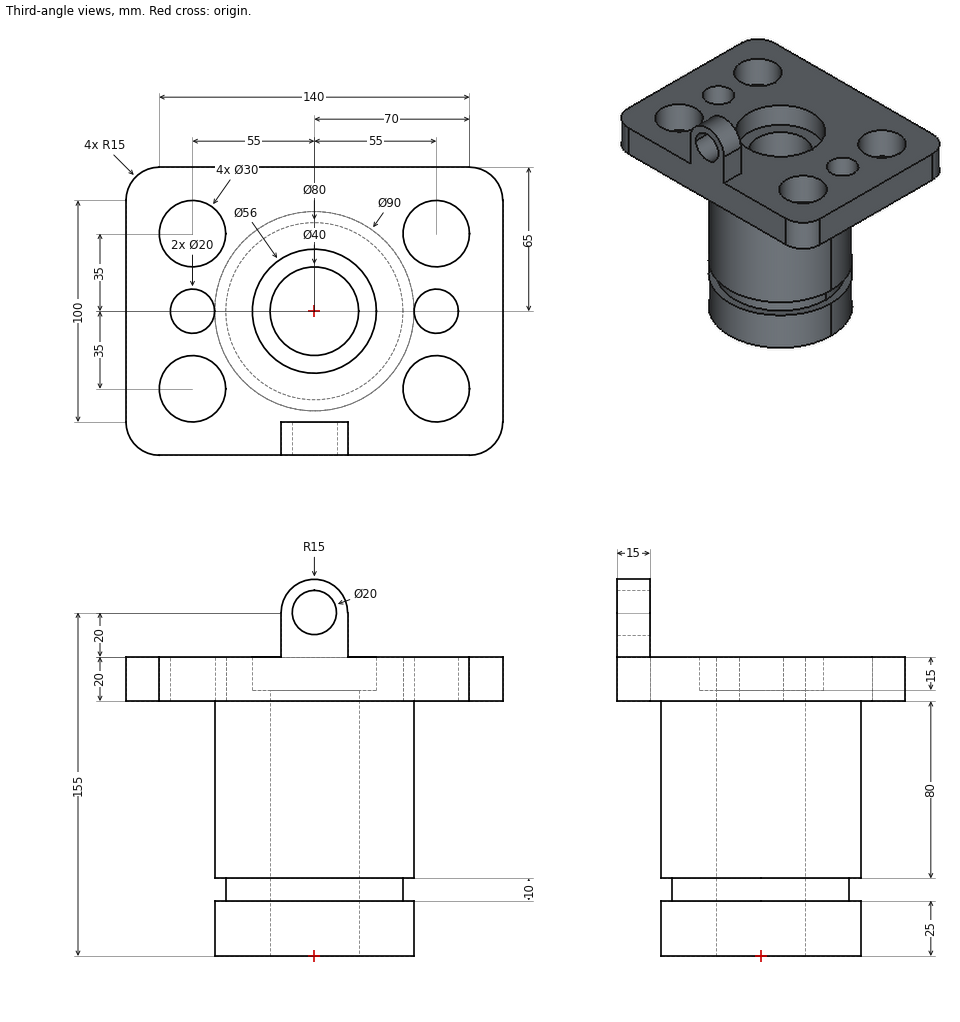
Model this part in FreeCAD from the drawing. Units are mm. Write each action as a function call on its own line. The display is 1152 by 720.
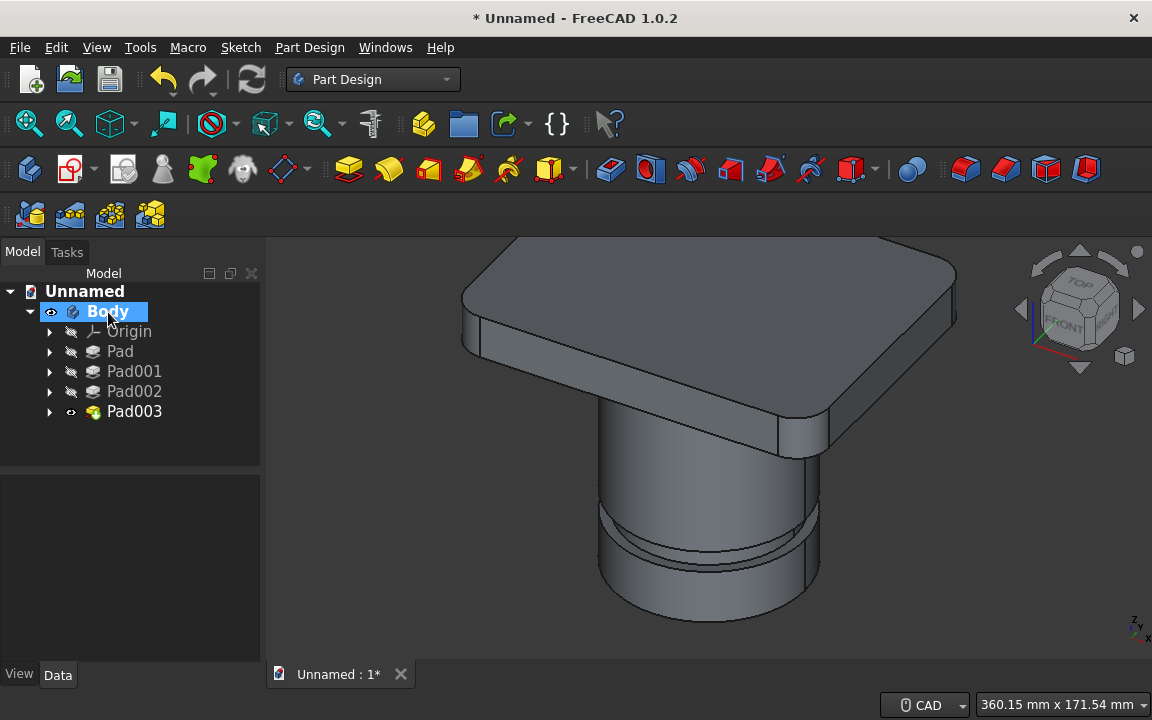
click(30, 124)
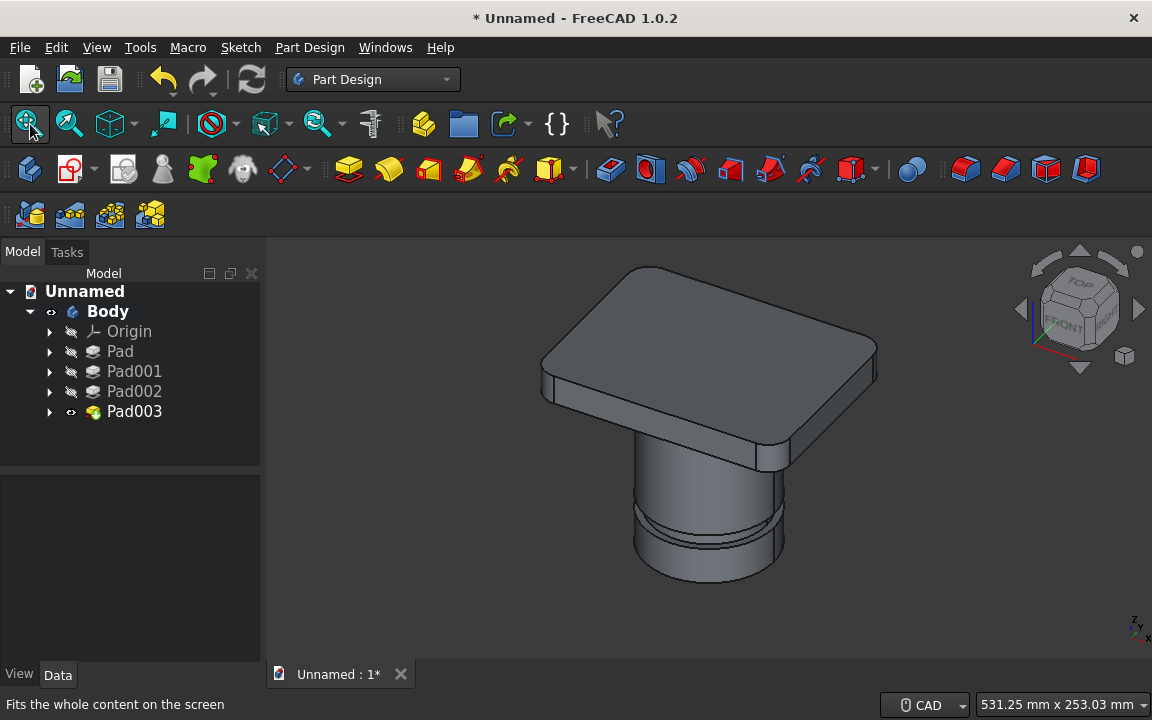
click(709, 355)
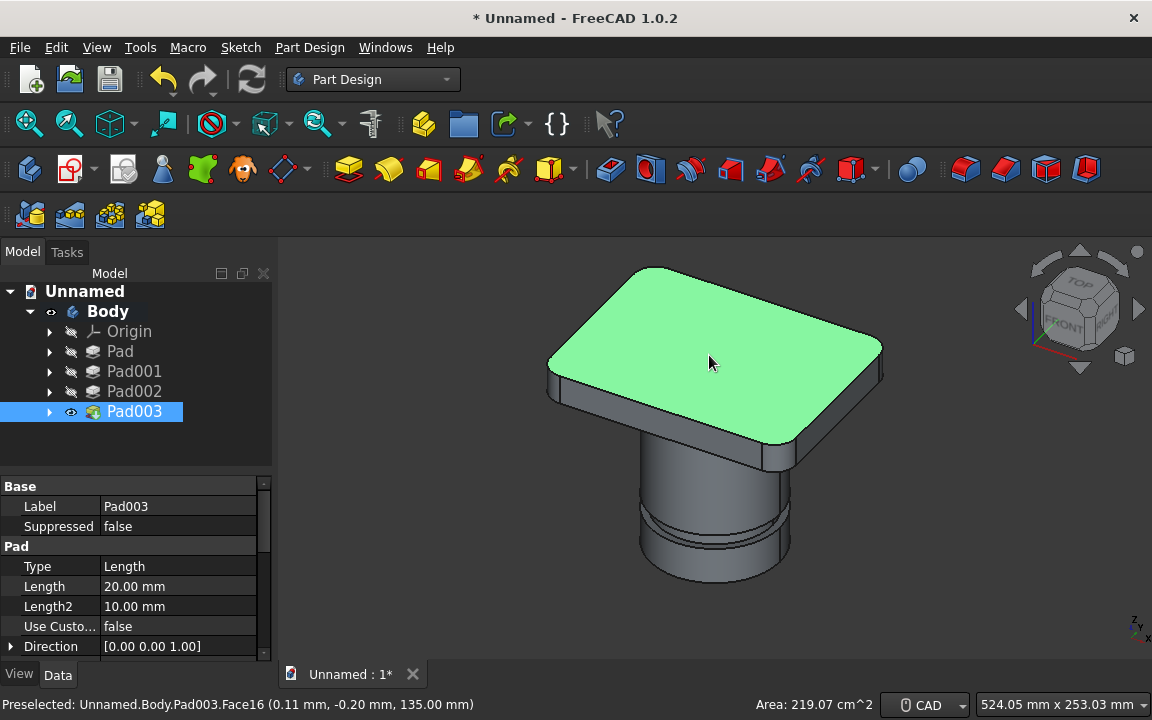
click(70, 170)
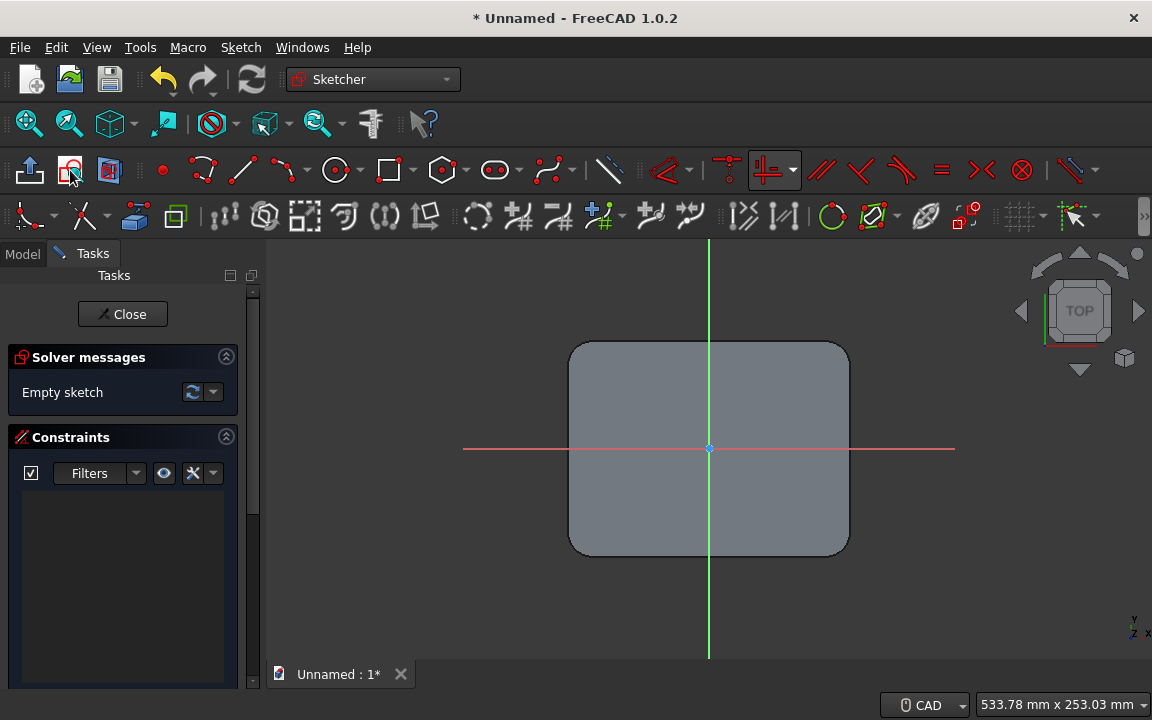
scroll(749, 449, up, 5)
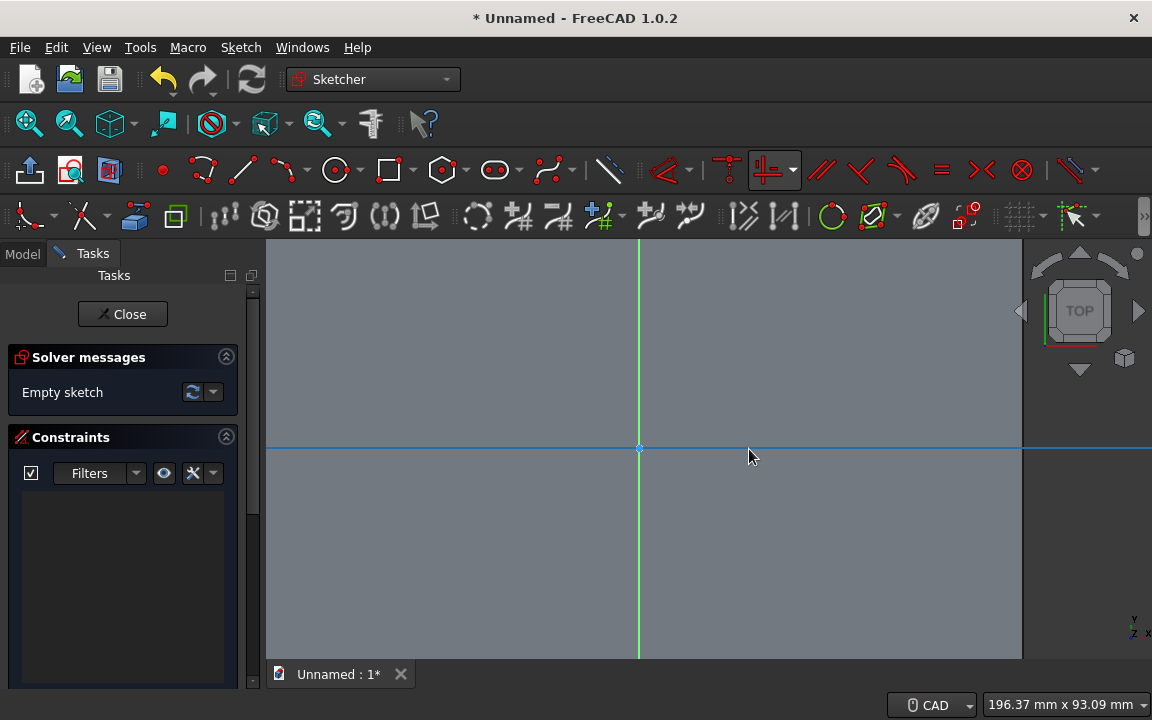
click(336, 170)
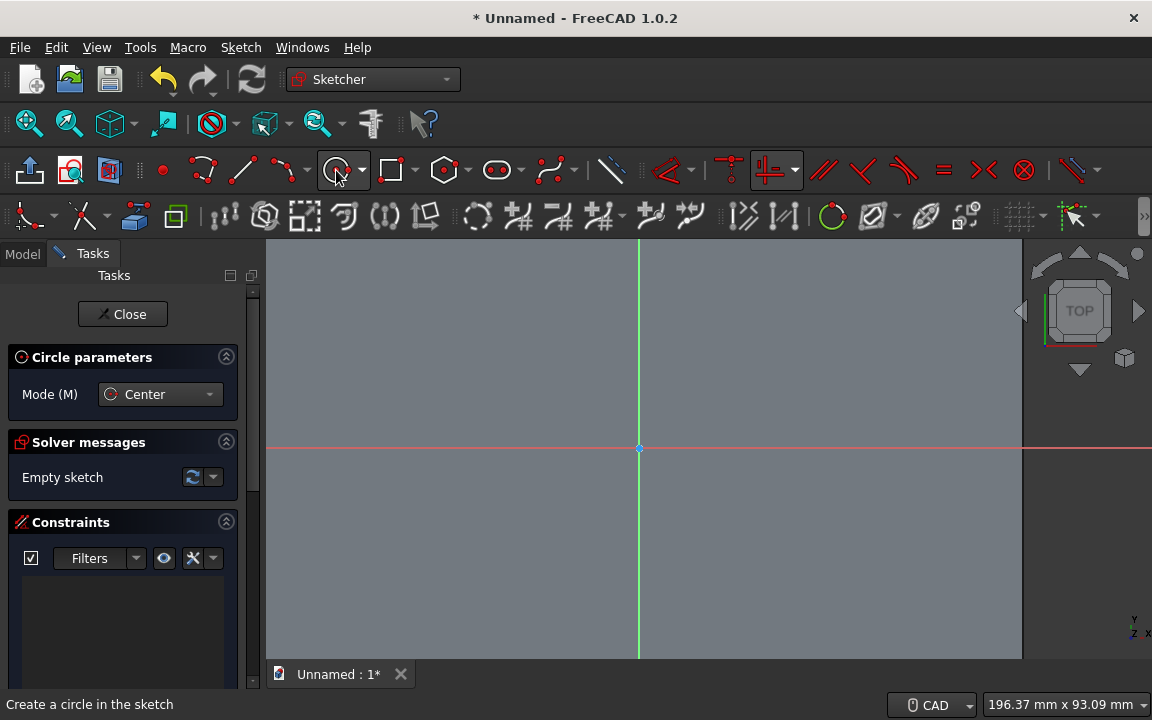
click(639, 448)
click(729, 359)
key(Escape)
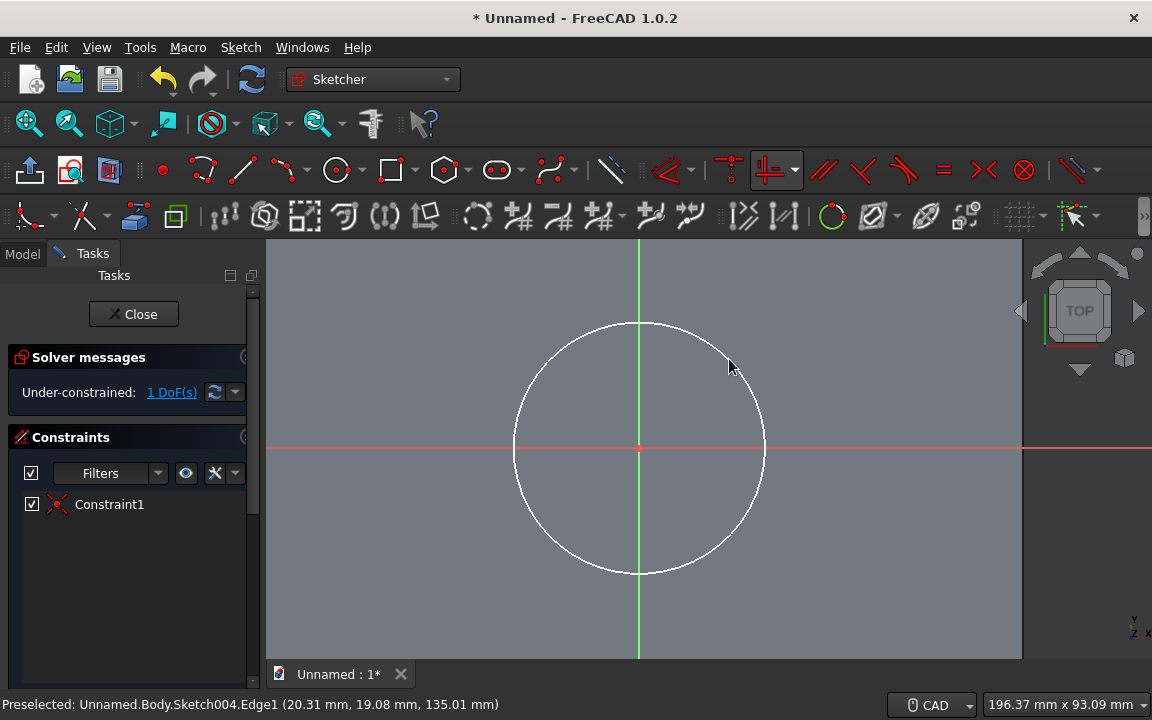
click(666, 170)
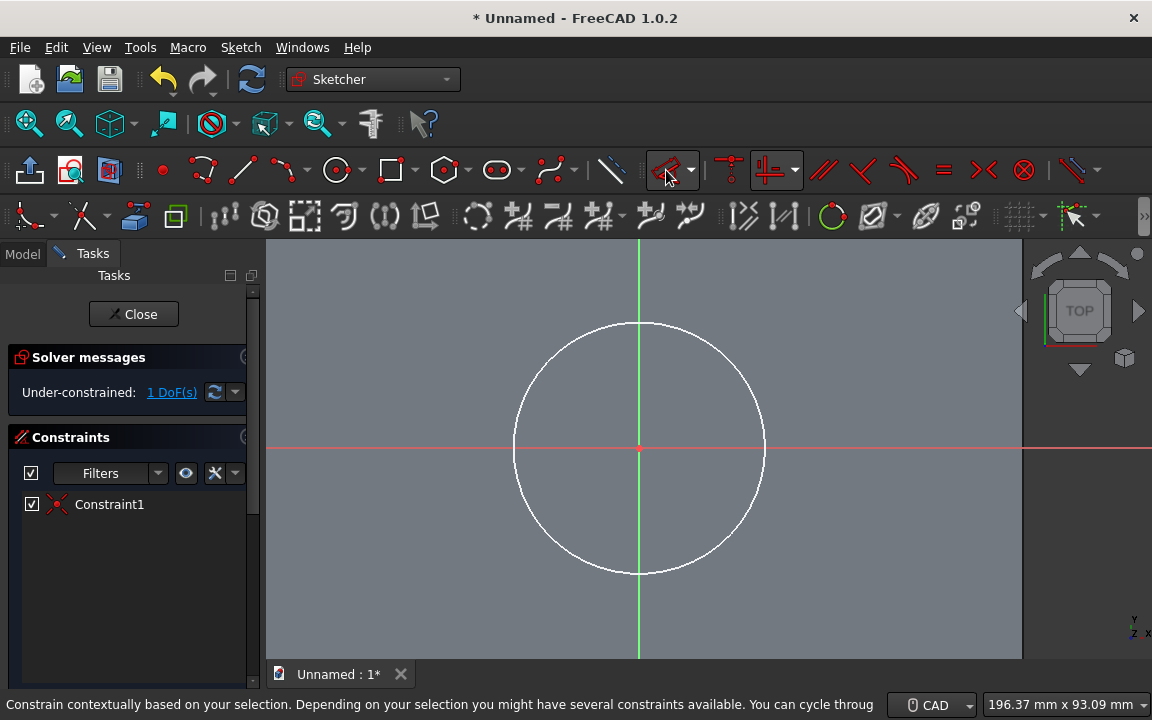
click(728, 359)
click(751, 336)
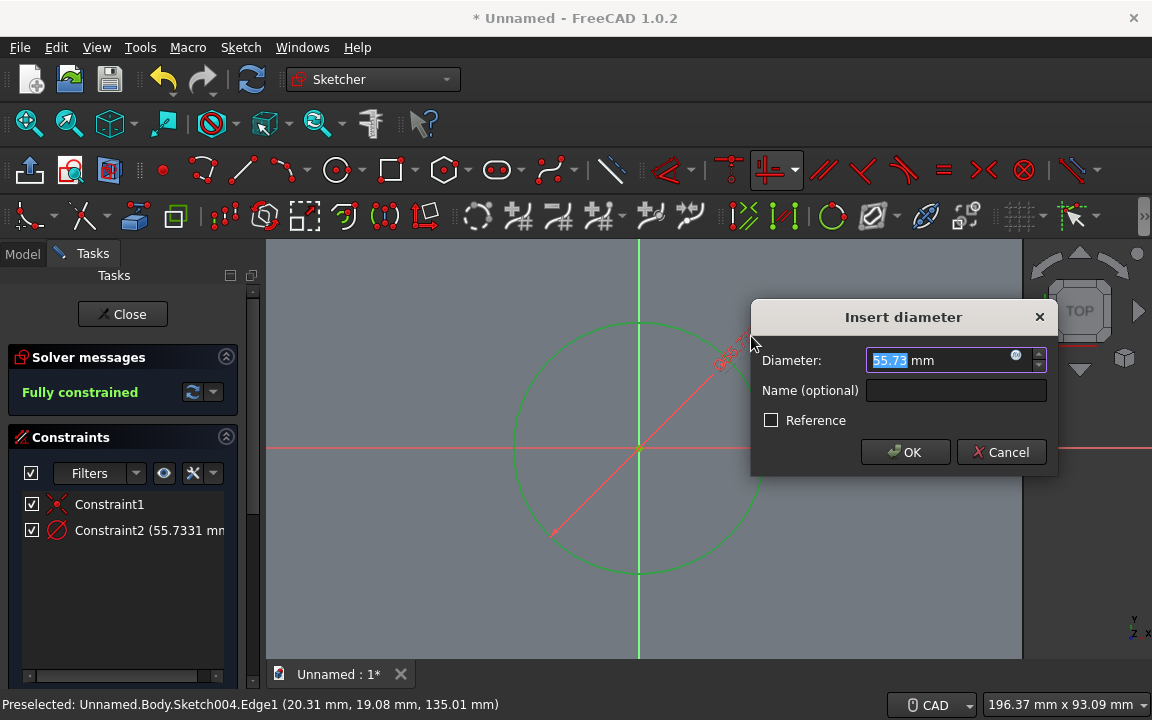
text(56)
key(Return)
key(Escape)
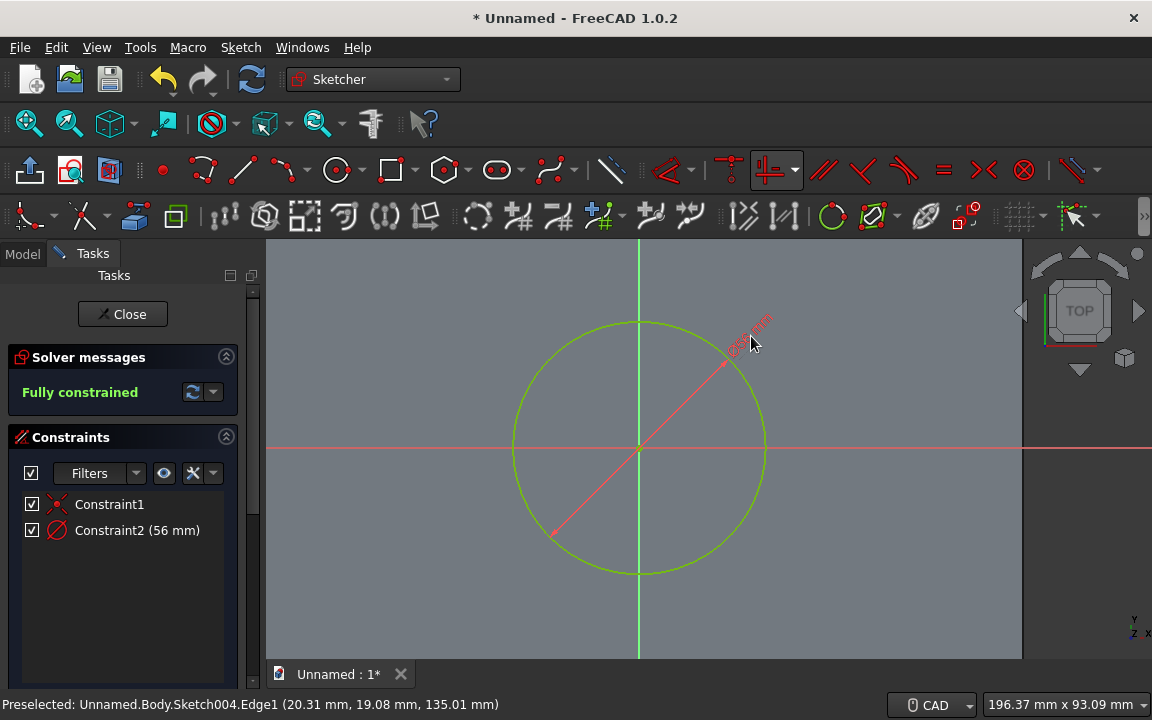
click(123, 314)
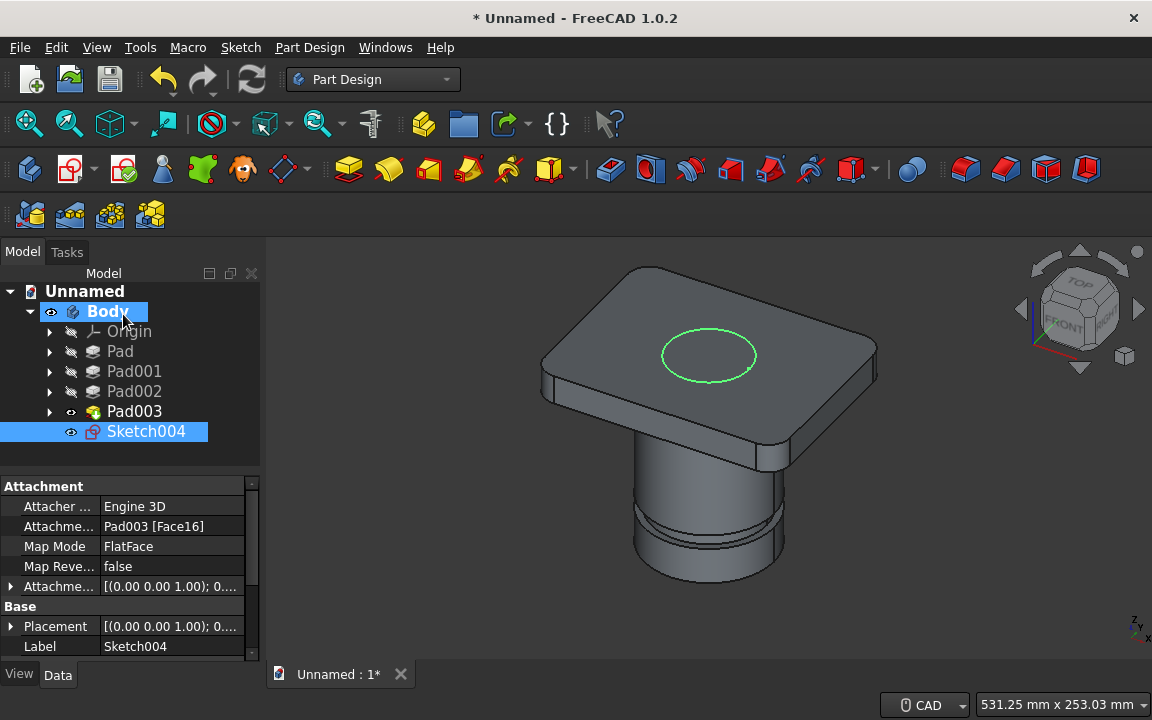
click(612, 170)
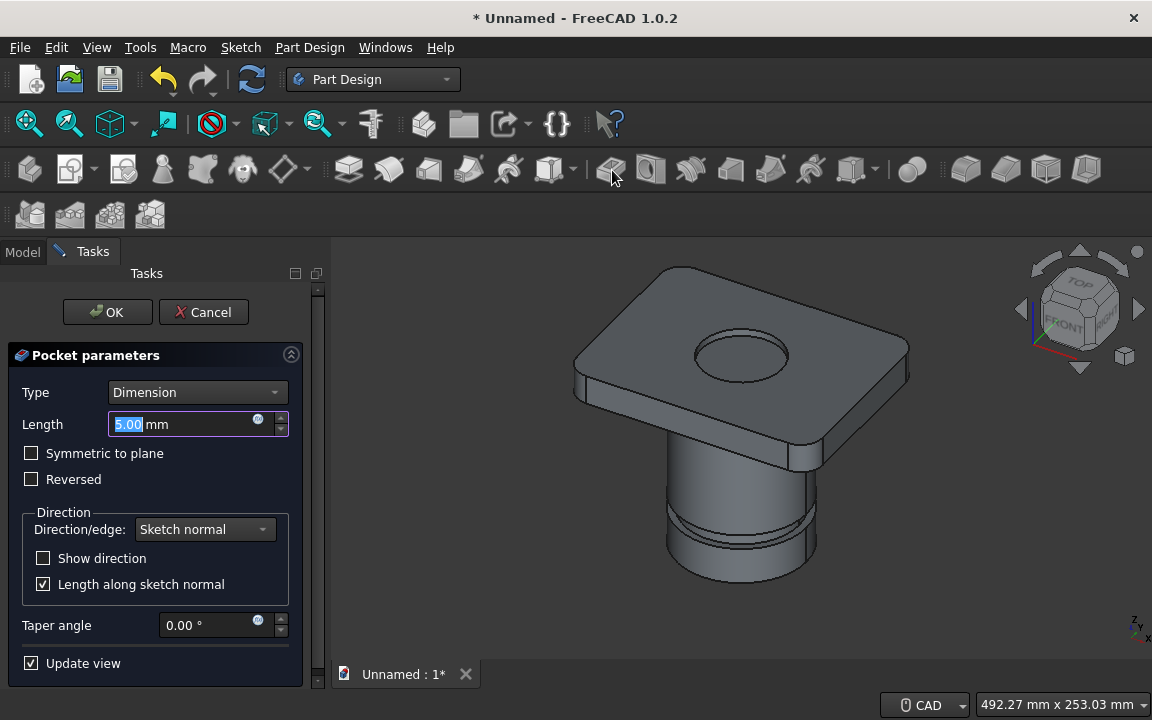
text(15)
key(Tab)